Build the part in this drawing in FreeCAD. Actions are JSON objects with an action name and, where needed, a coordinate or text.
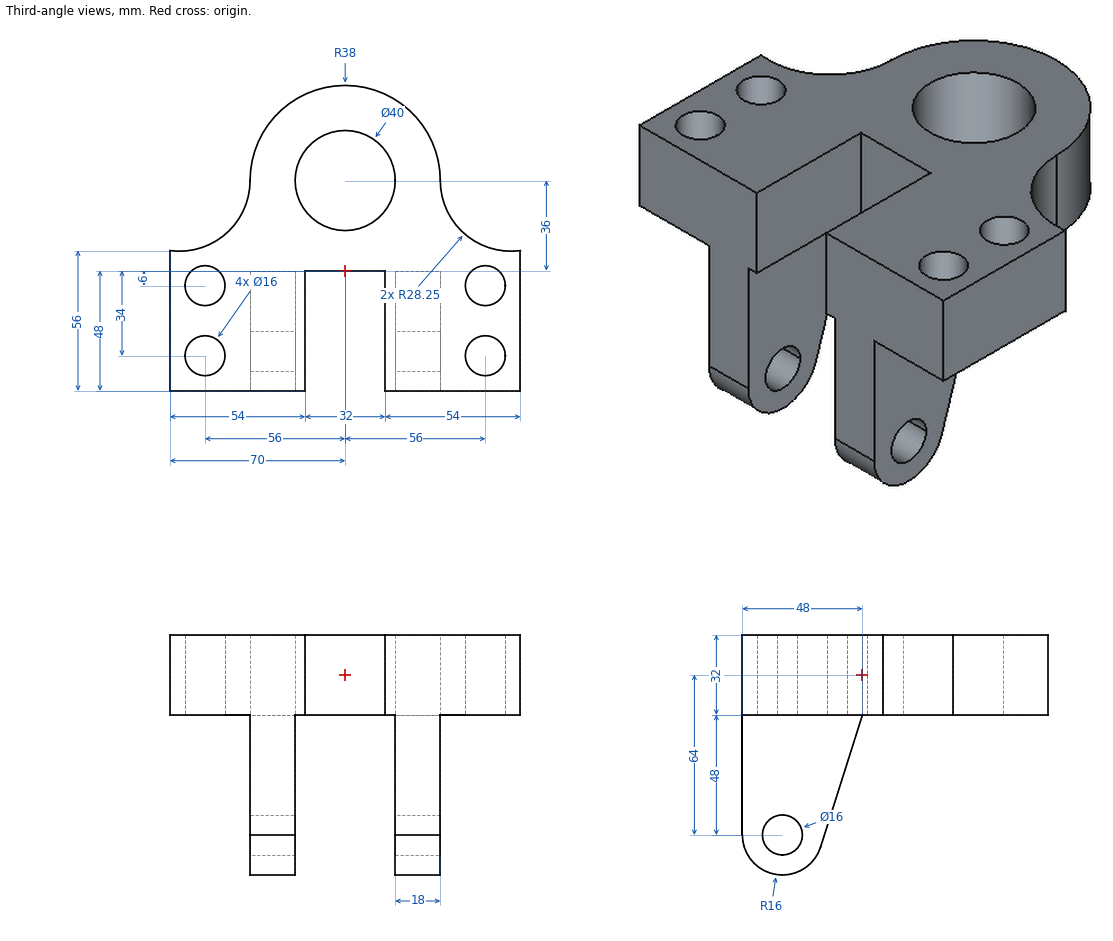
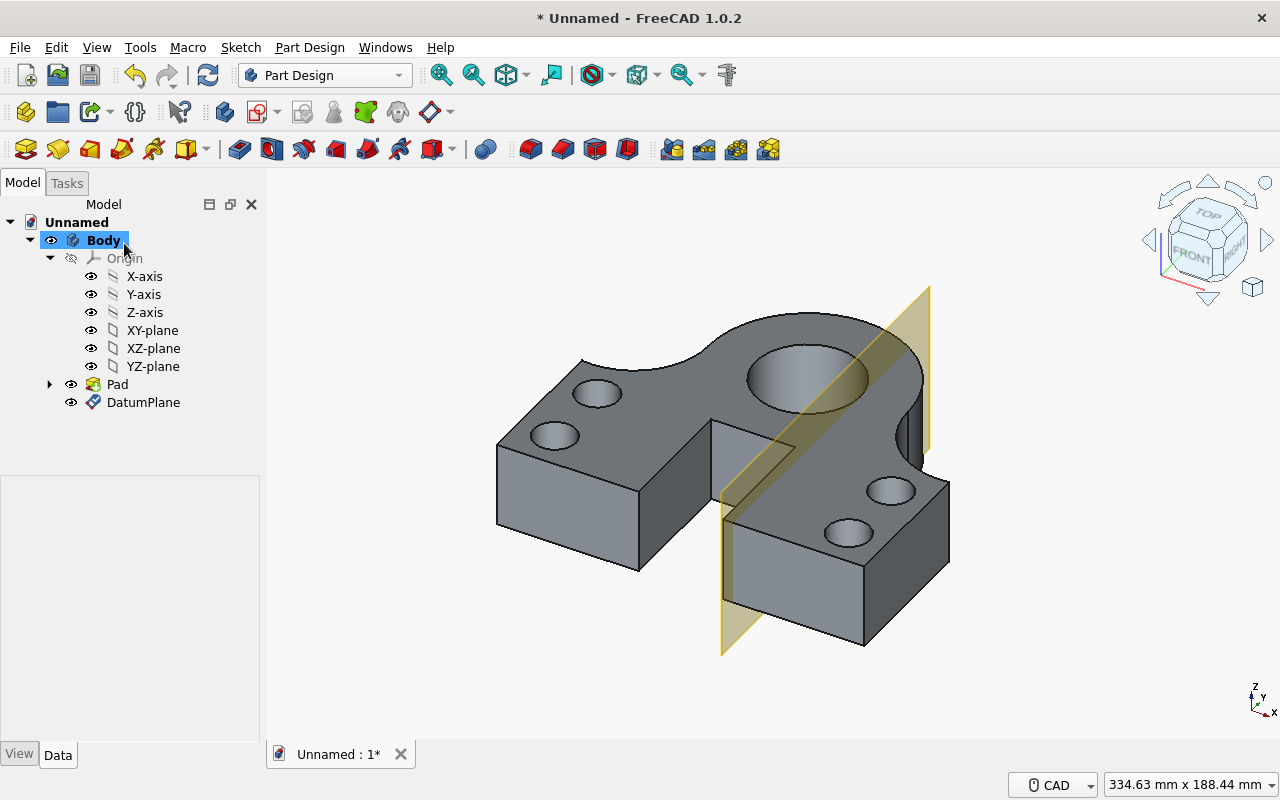
{"action": "left_click", "coordinate": [116, 402]}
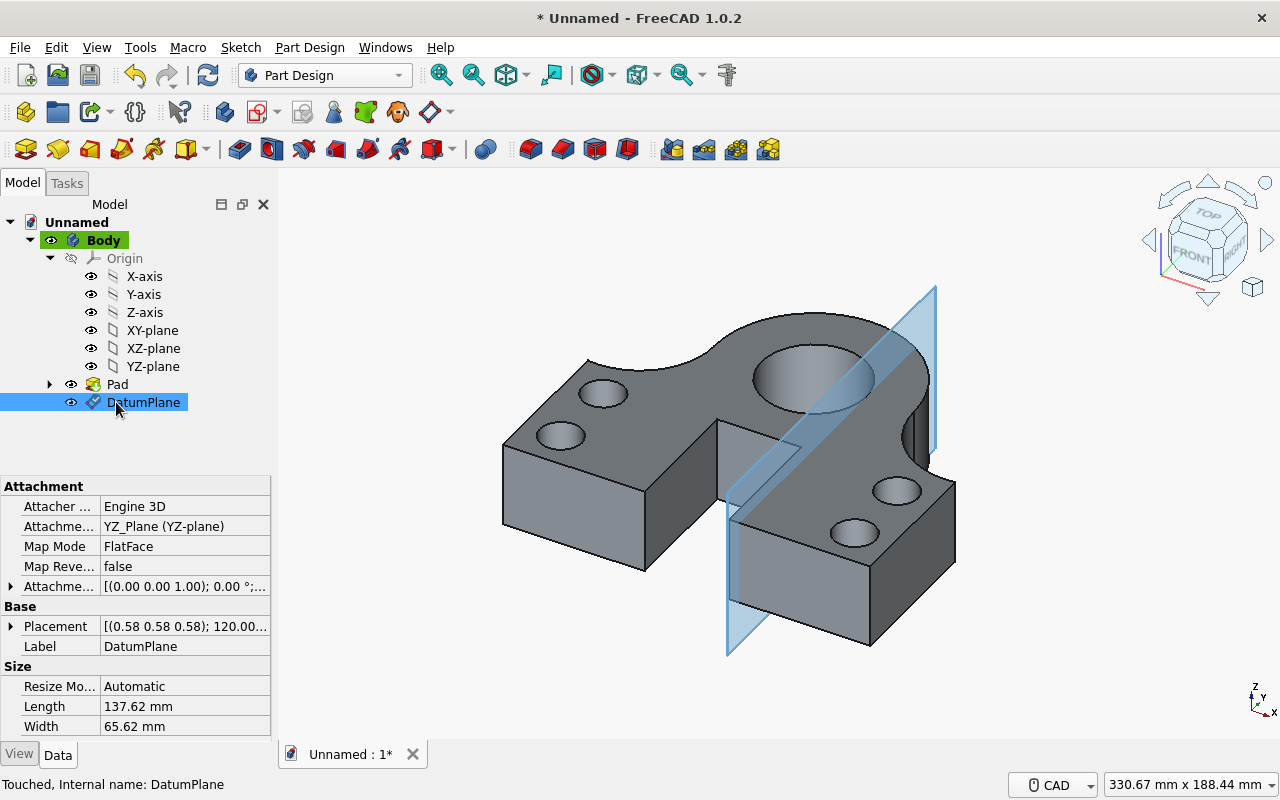
{"action": "left_click", "coordinate": [258, 112]}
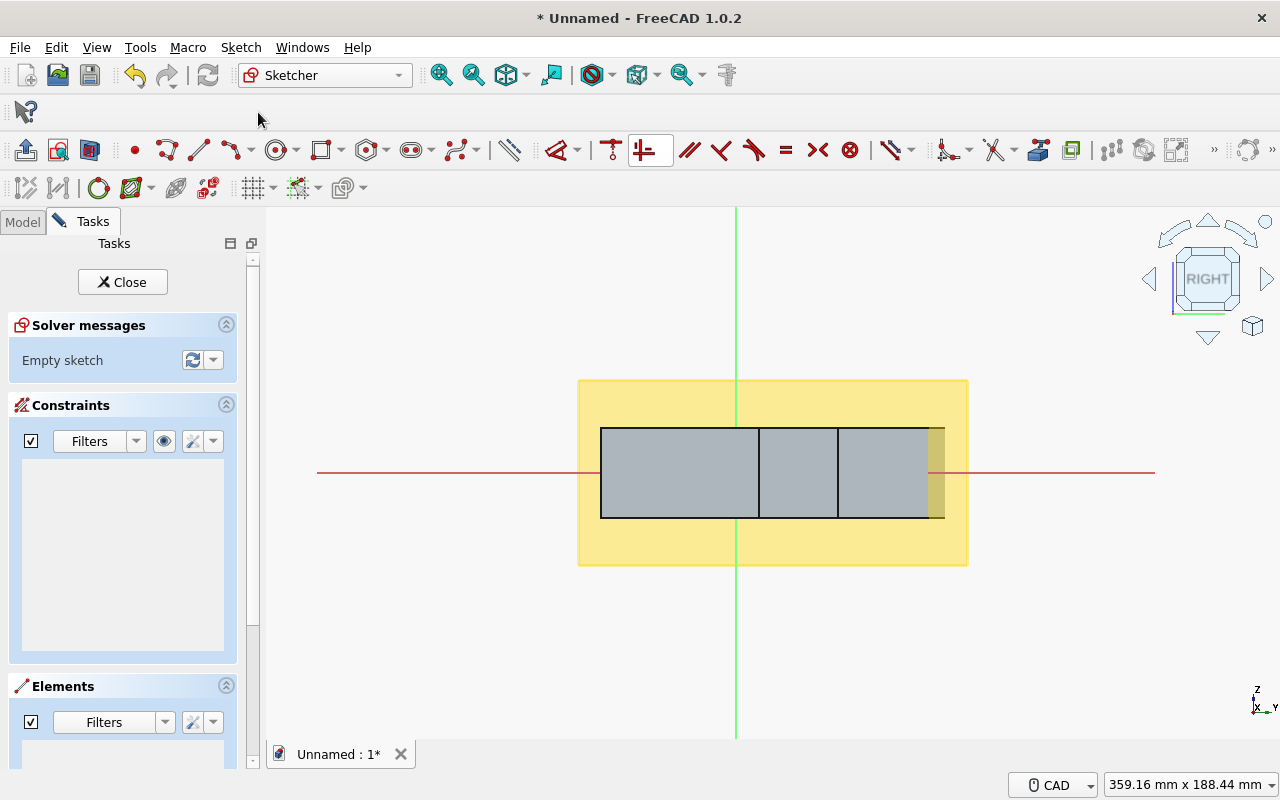
{"action": "left_click", "coordinate": [90, 150]}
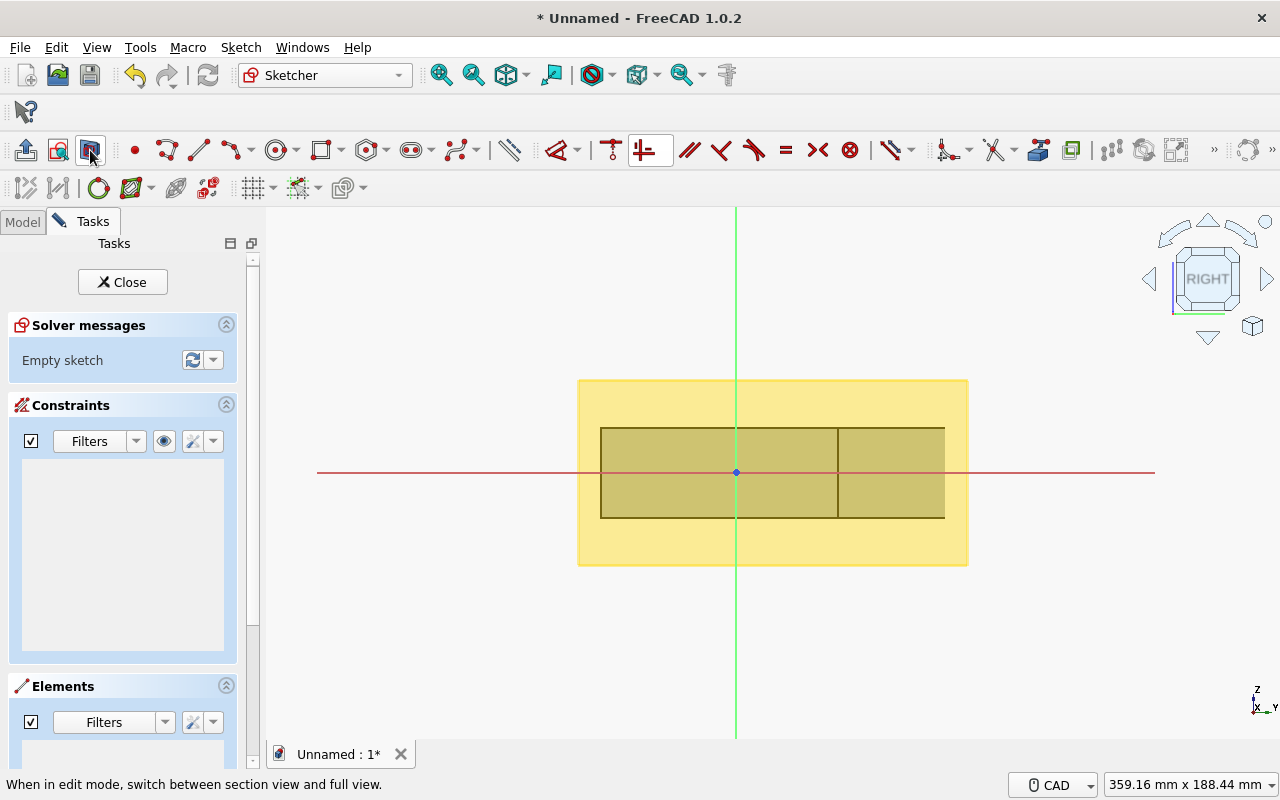
{"action": "scroll", "coordinate": [867, 235], "scroll_direction": "down", "scroll_amount": 1}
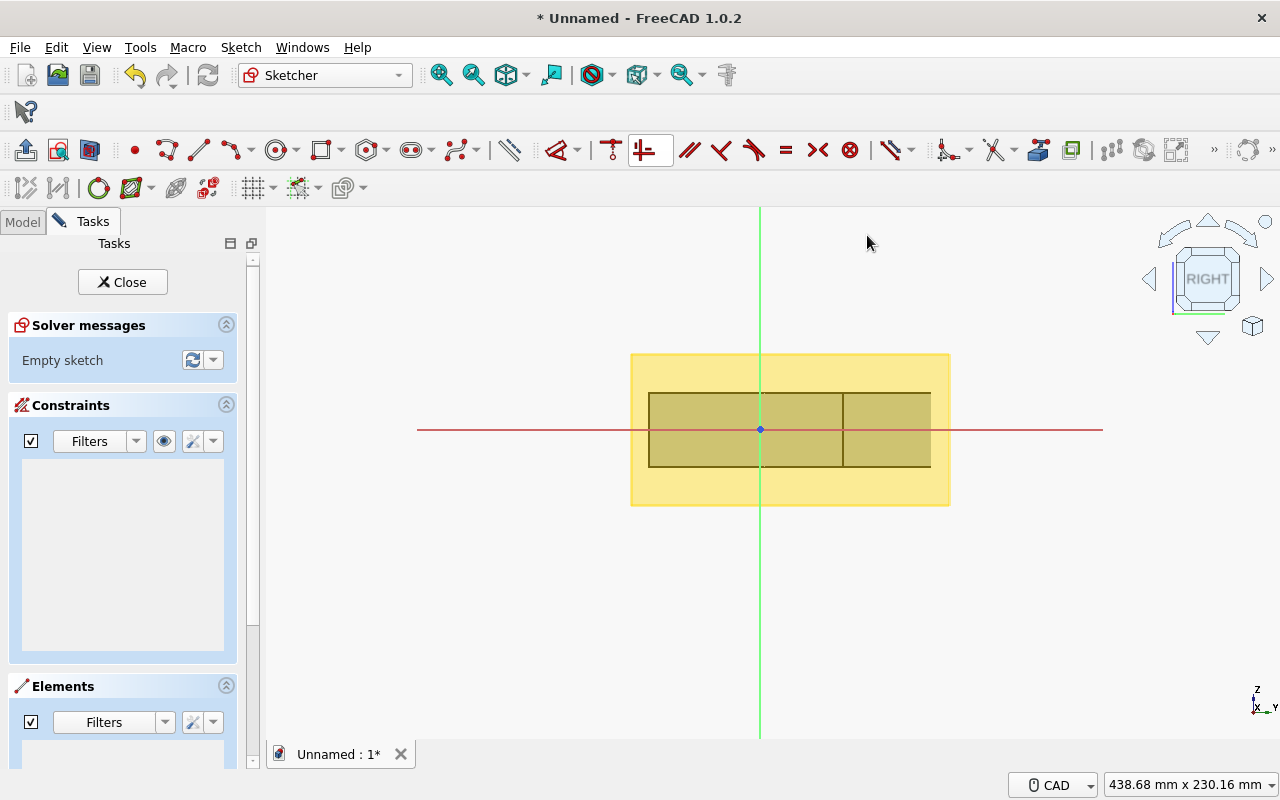
{"action": "scroll", "coordinate": [705, 582], "scroll_direction": "up", "scroll_amount": 3}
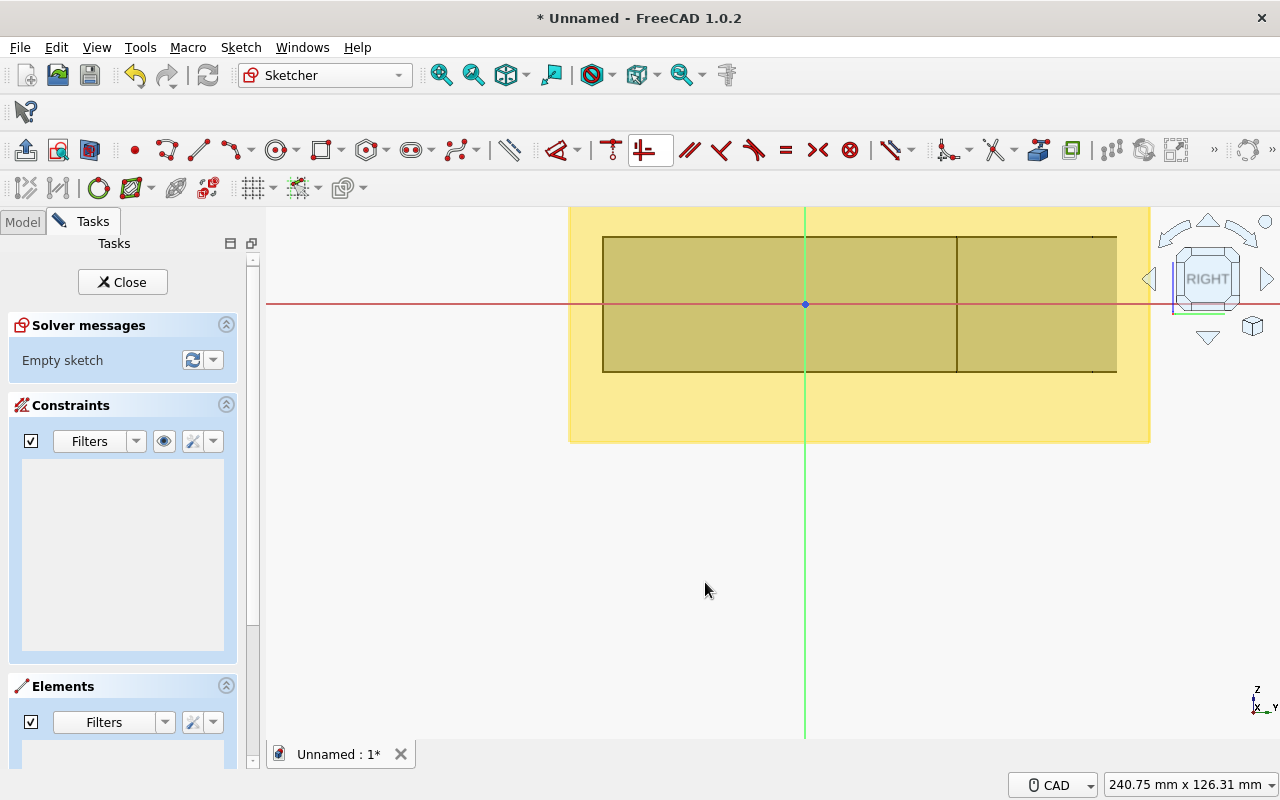
{"action": "left_click", "coordinate": [168, 150]}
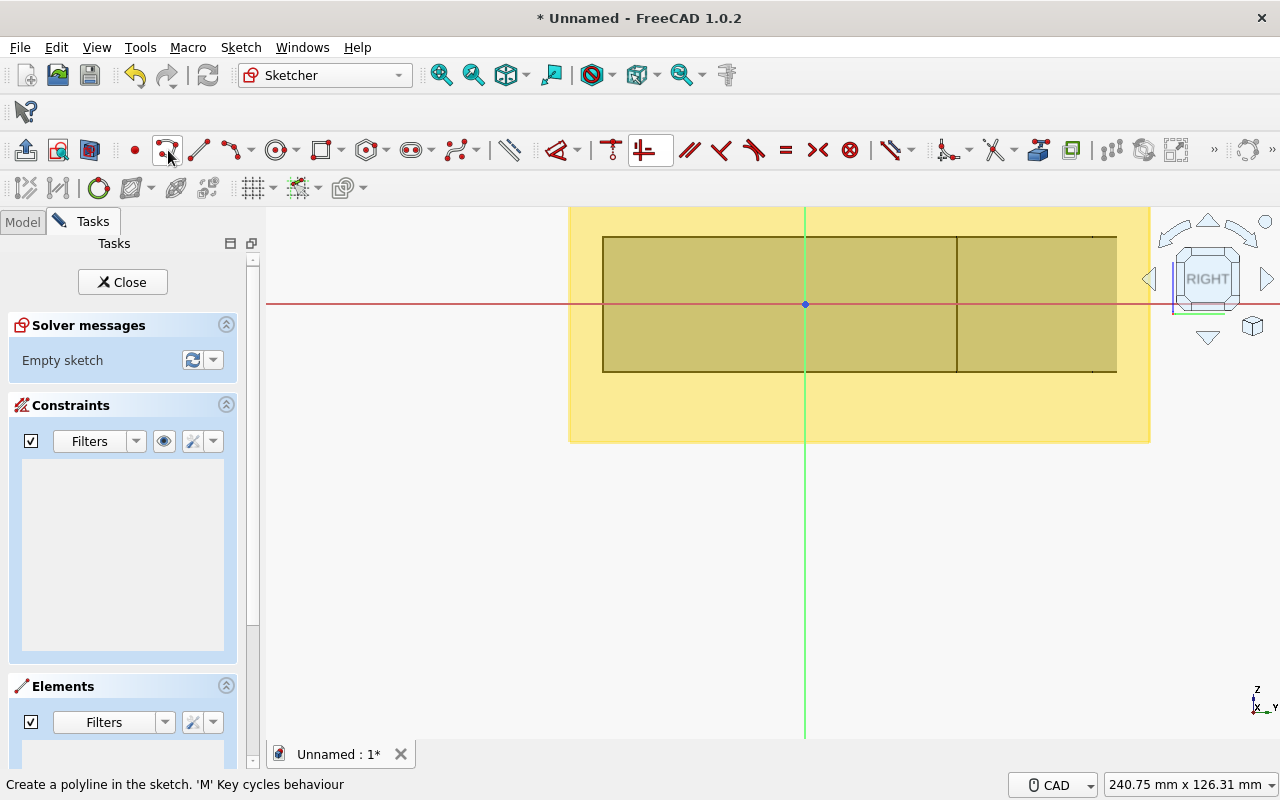
{"action": "left_click", "coordinate": [734, 594]}
{"action": "left_click", "coordinate": [805, 372]}
{"action": "left_click", "coordinate": [603, 372]}
{"action": "left_click", "coordinate": [603, 574]}
{"action": "right_click", "coordinate": [603, 574]}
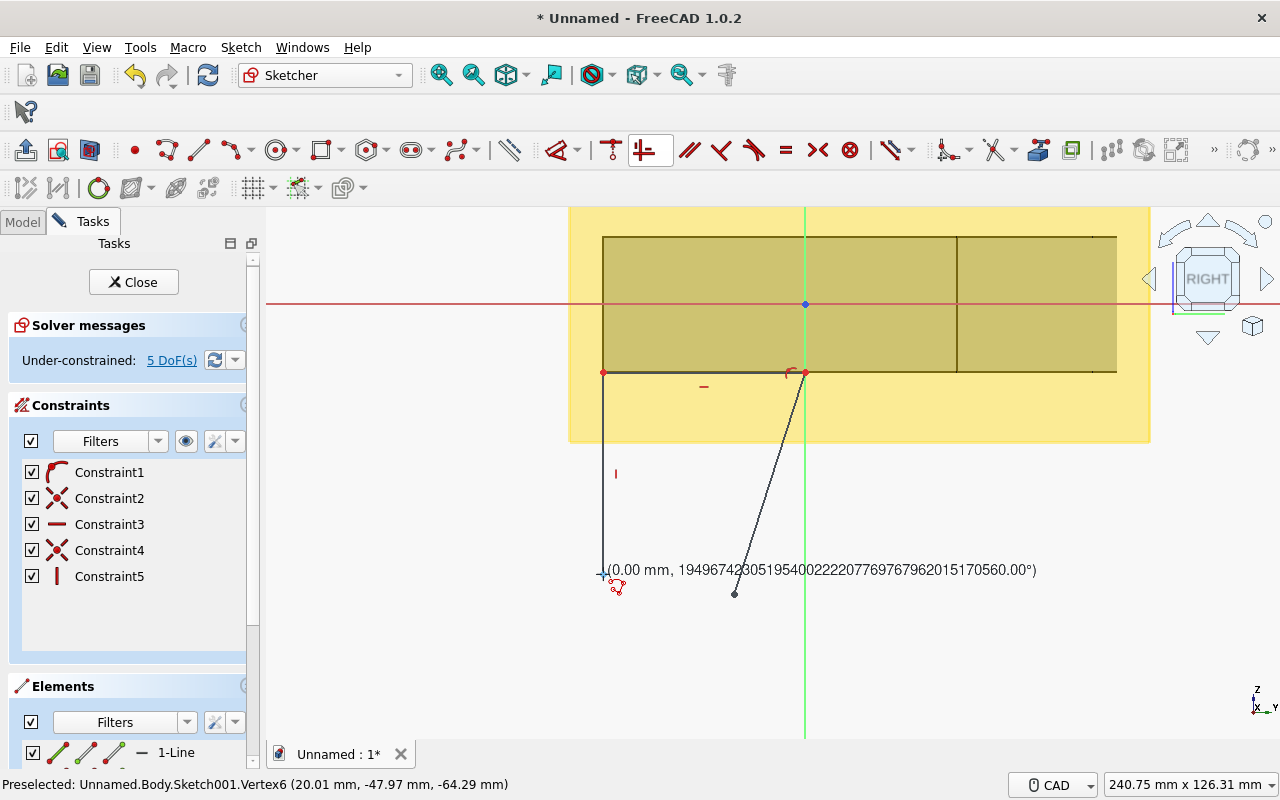
{"action": "left_click", "coordinate": [232, 150]}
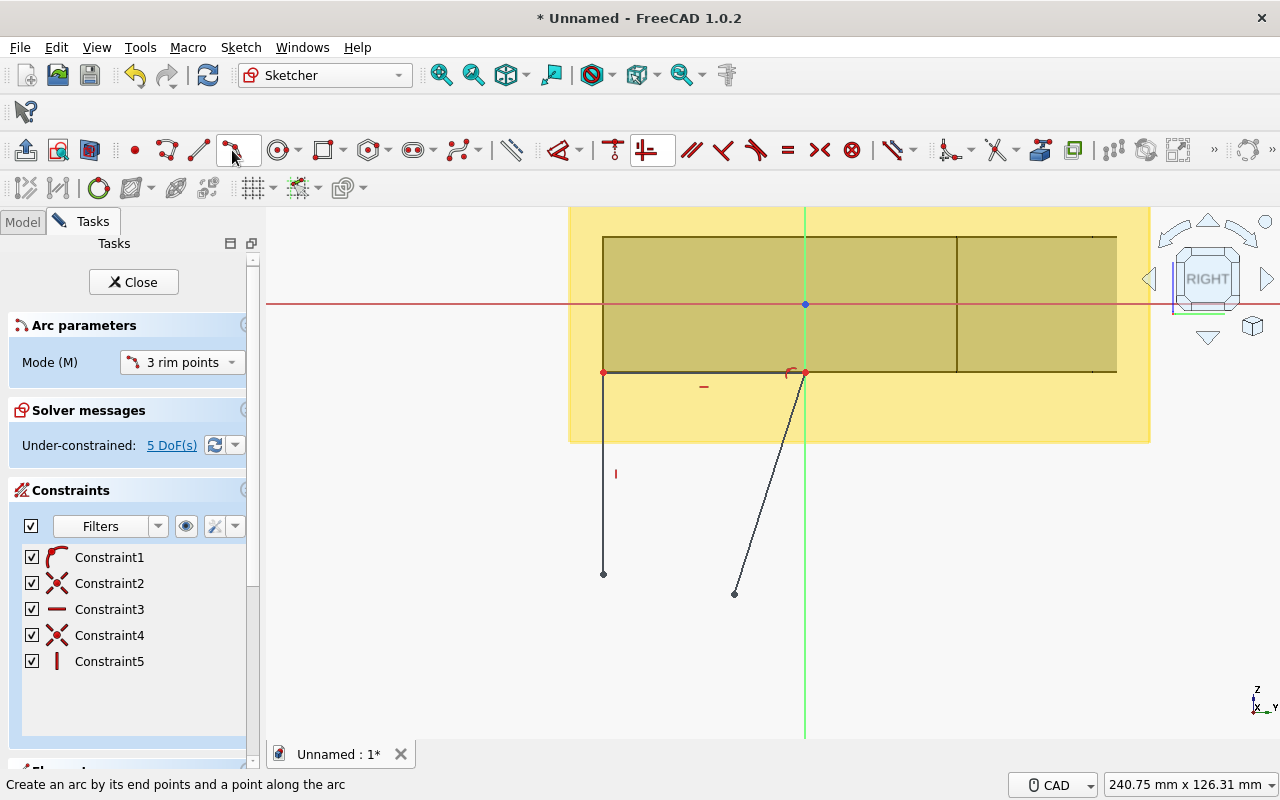
{"action": "left_click", "coordinate": [603, 575]}
{"action": "left_click", "coordinate": [734, 595]}
{"action": "left_click", "coordinate": [660, 640]}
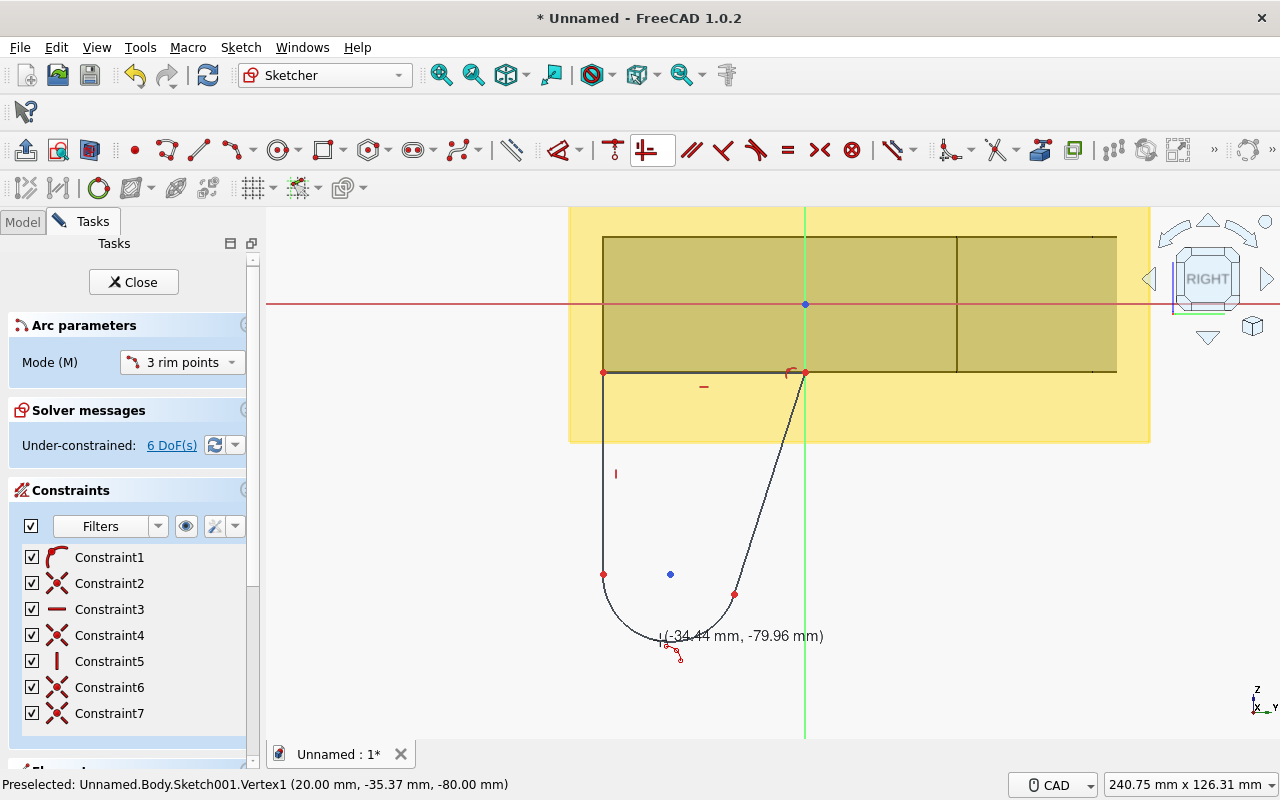
{"action": "left_click", "coordinate": [278, 150]}